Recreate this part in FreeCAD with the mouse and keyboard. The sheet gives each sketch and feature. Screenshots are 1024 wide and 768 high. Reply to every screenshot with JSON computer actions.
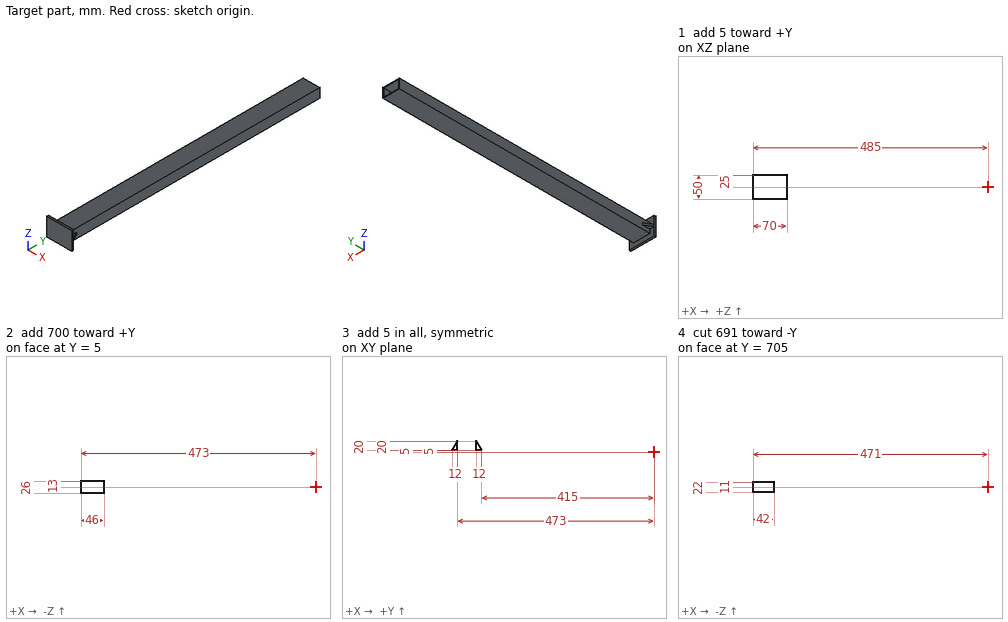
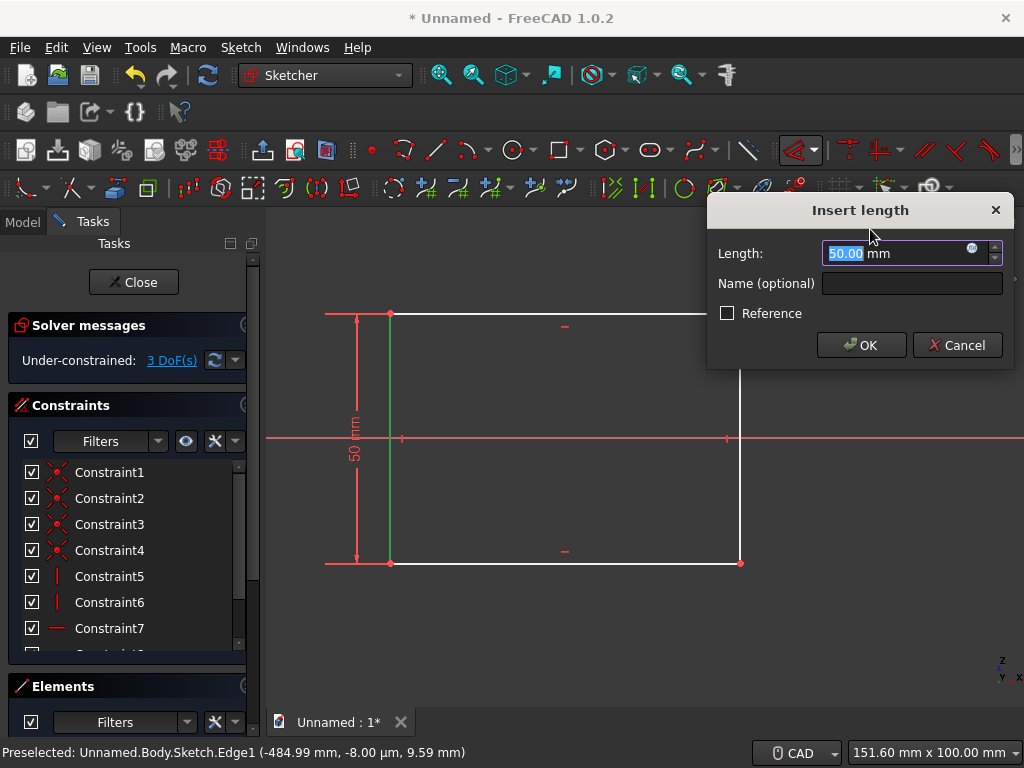
{"action": "type", "text": "50"}
{"action": "key", "text": "Return"}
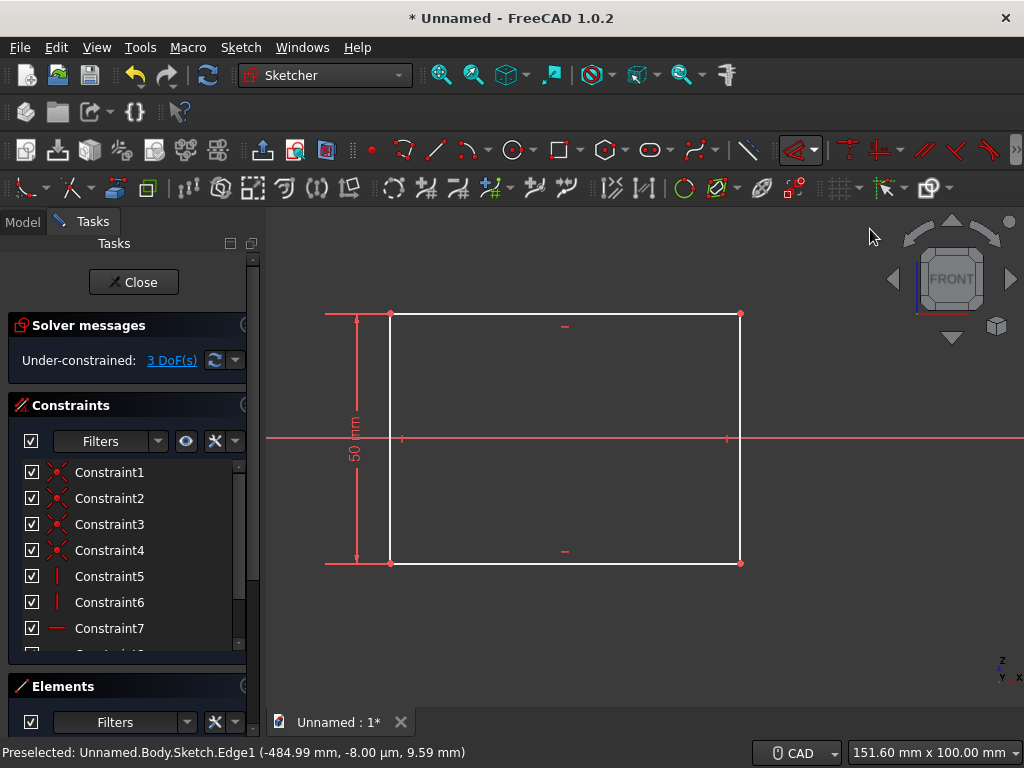
{"action": "left_click", "coordinate": [495, 564]}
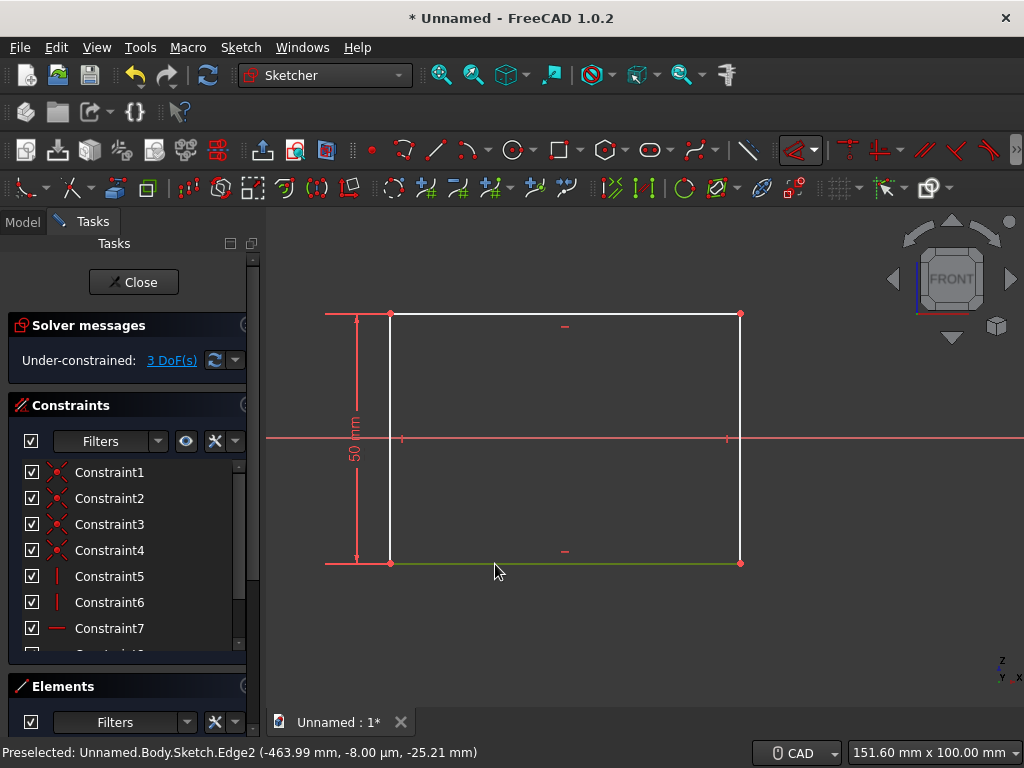
{"action": "key", "text": "l"}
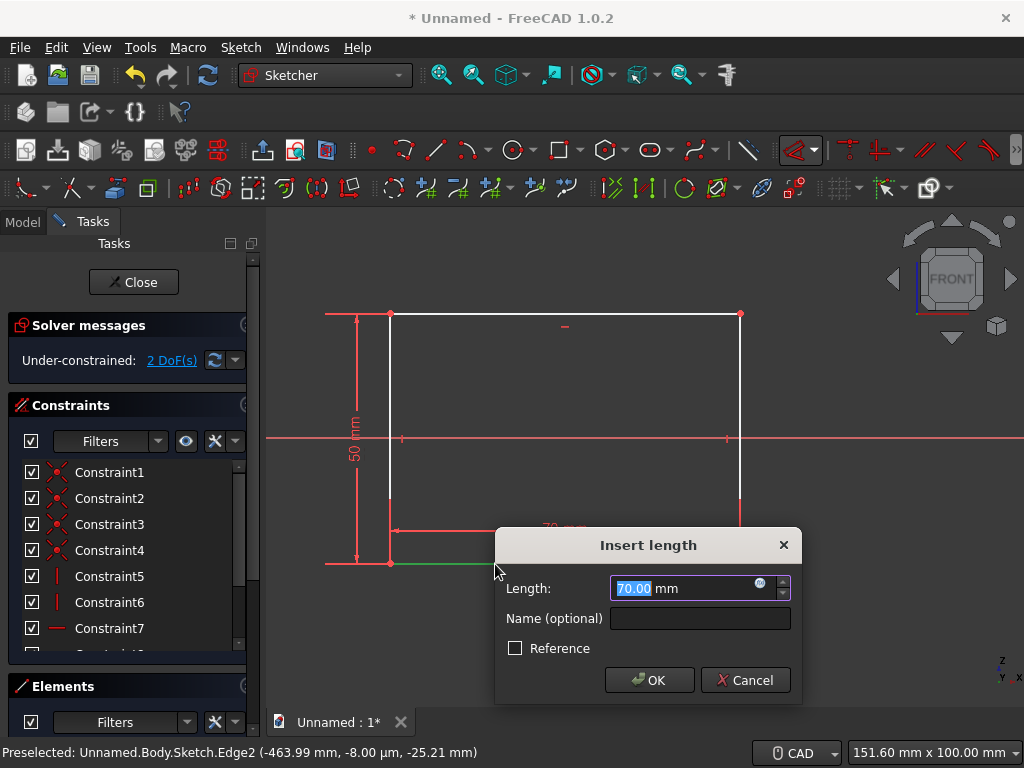
{"action": "type", "text": "70"}
{"action": "key", "text": "Return"}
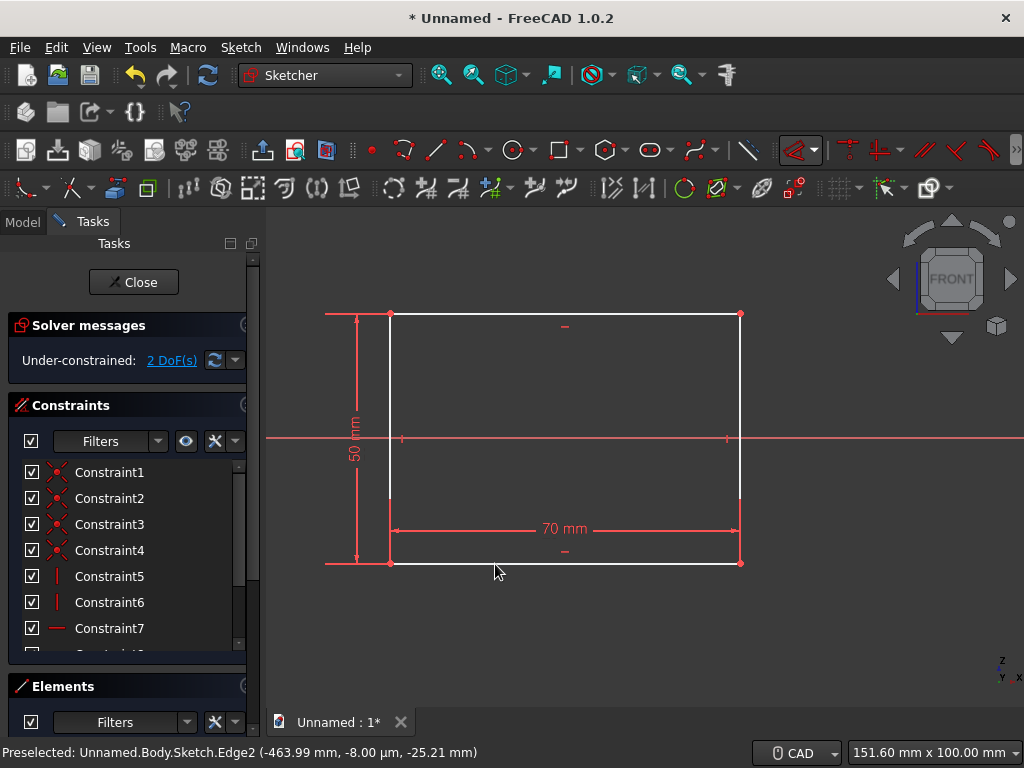
{"action": "left_click", "coordinate": [390, 314]}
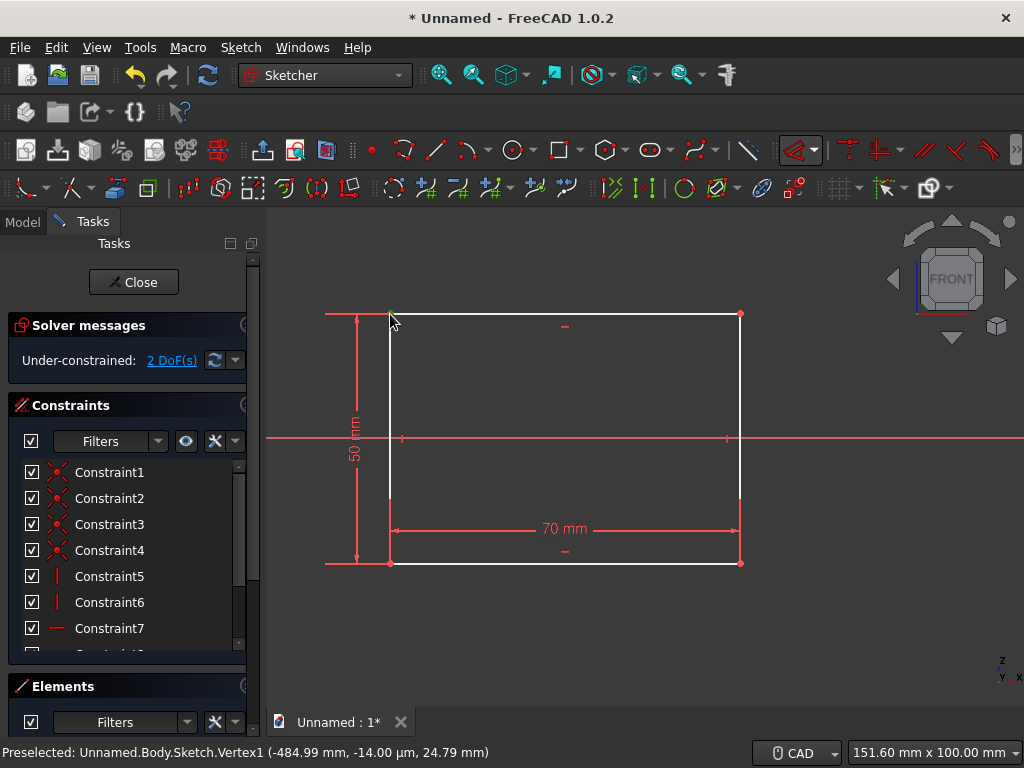
{"action": "left_click", "coordinate": [816, 150]}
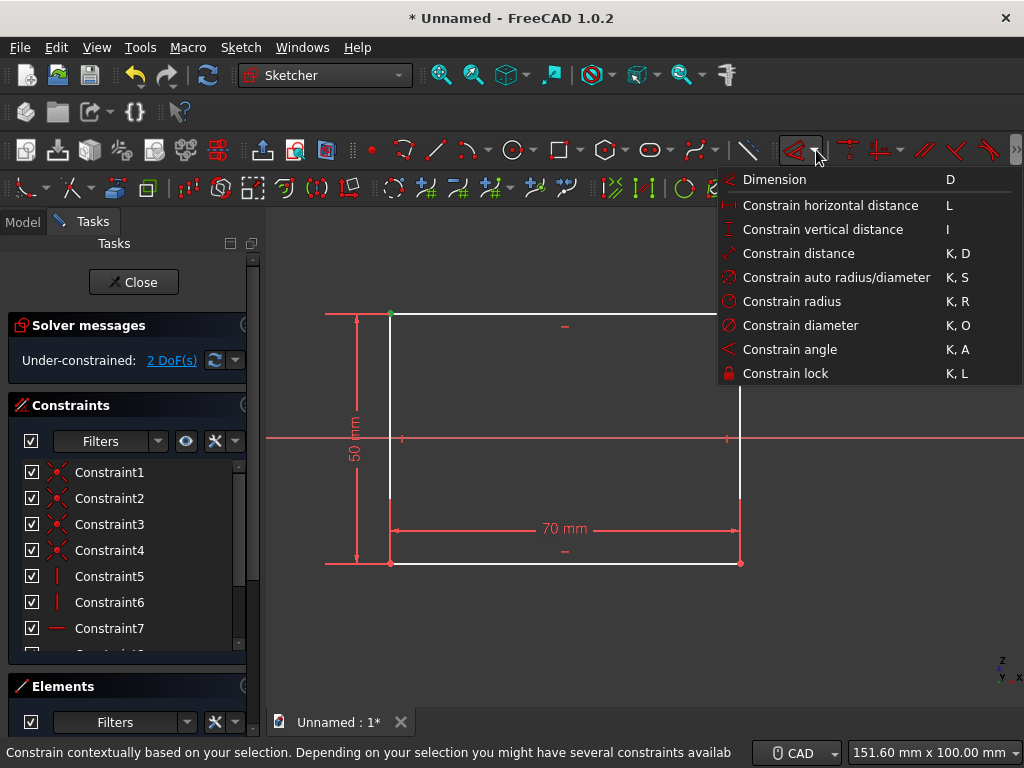
{"action": "left_click", "coordinate": [870, 229]}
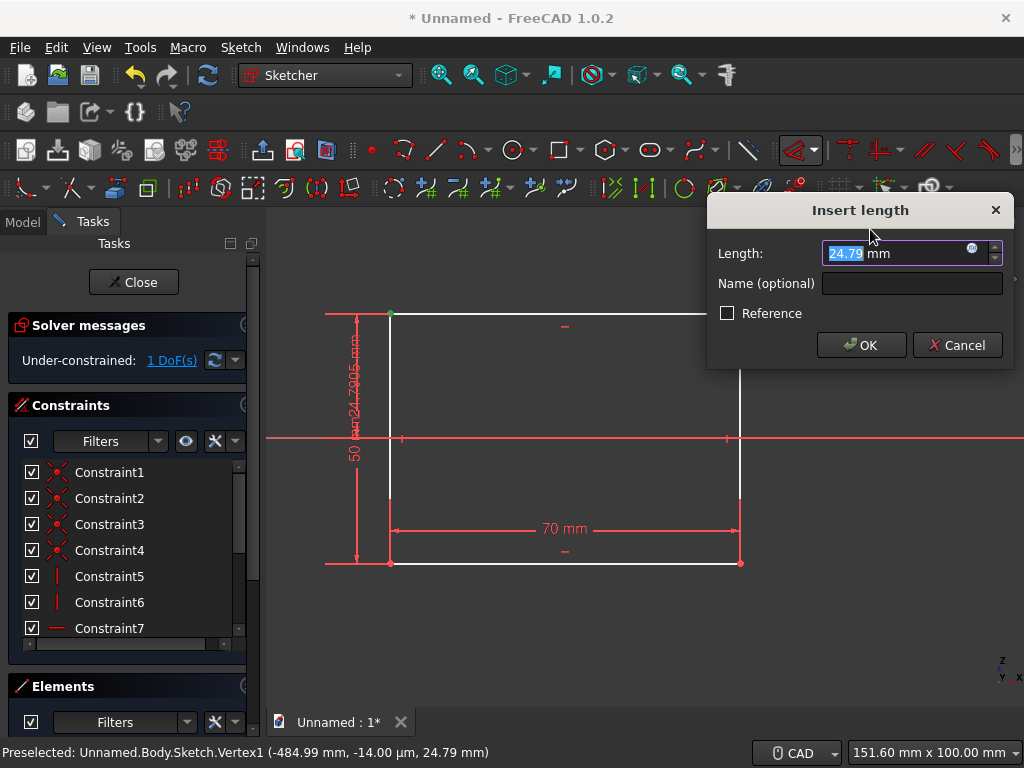
{"action": "type", "text": "25"}
{"action": "key", "text": "Return"}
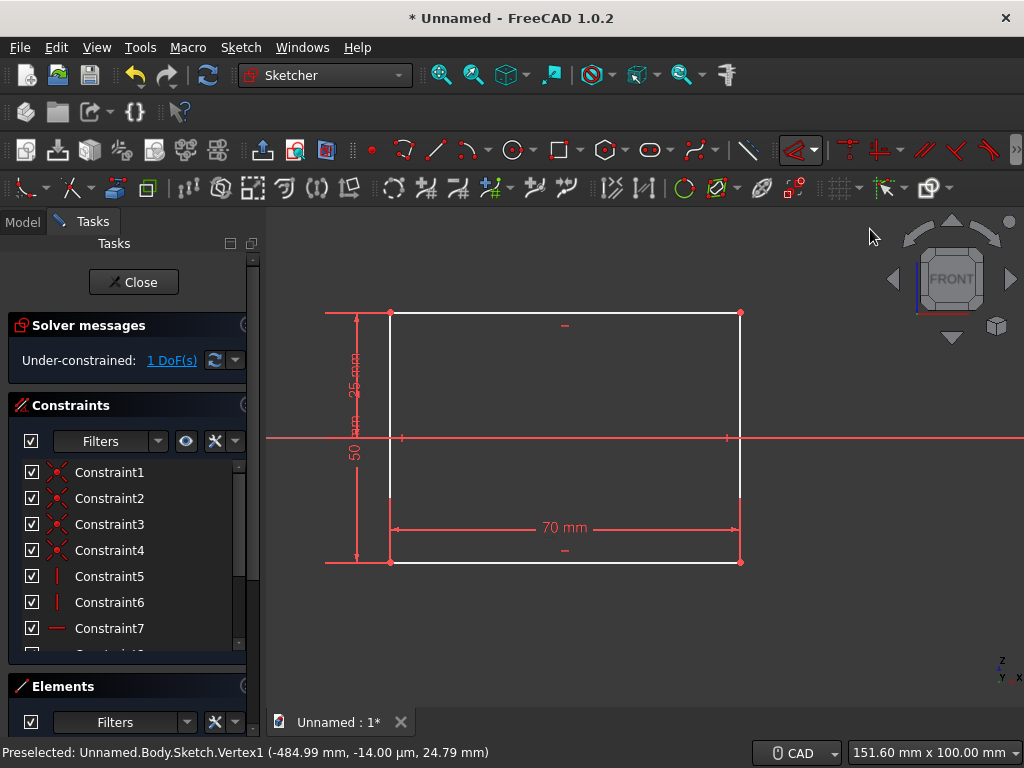
{"action": "left_click", "coordinate": [390, 313]}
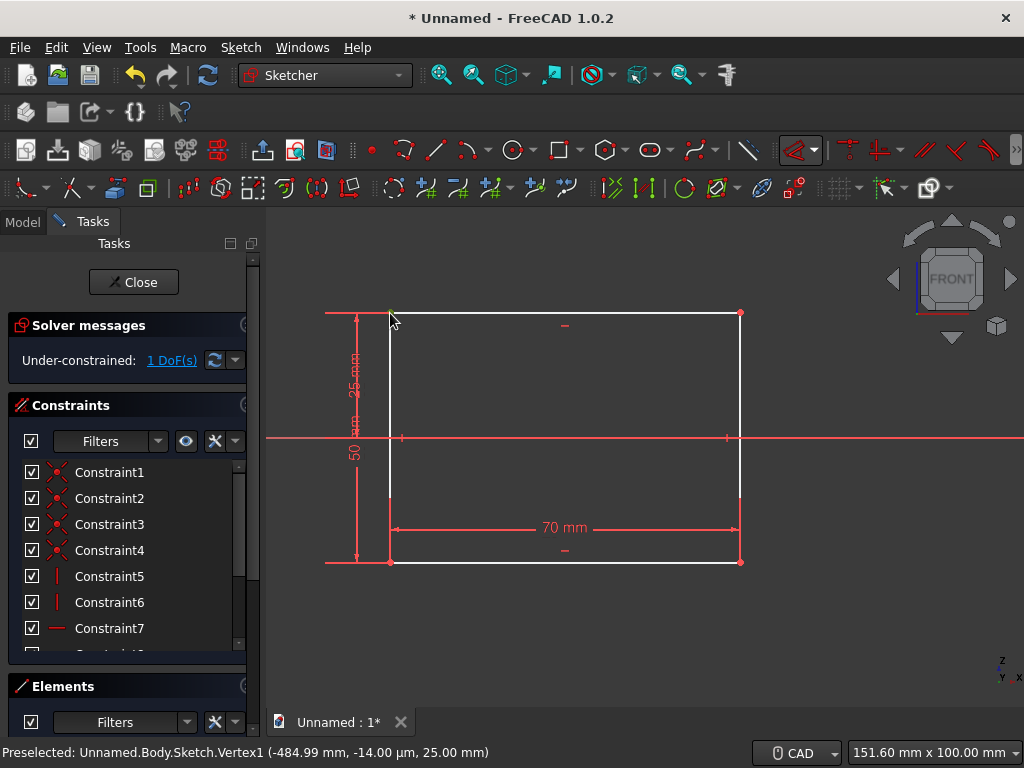
{"action": "key", "text": "l"}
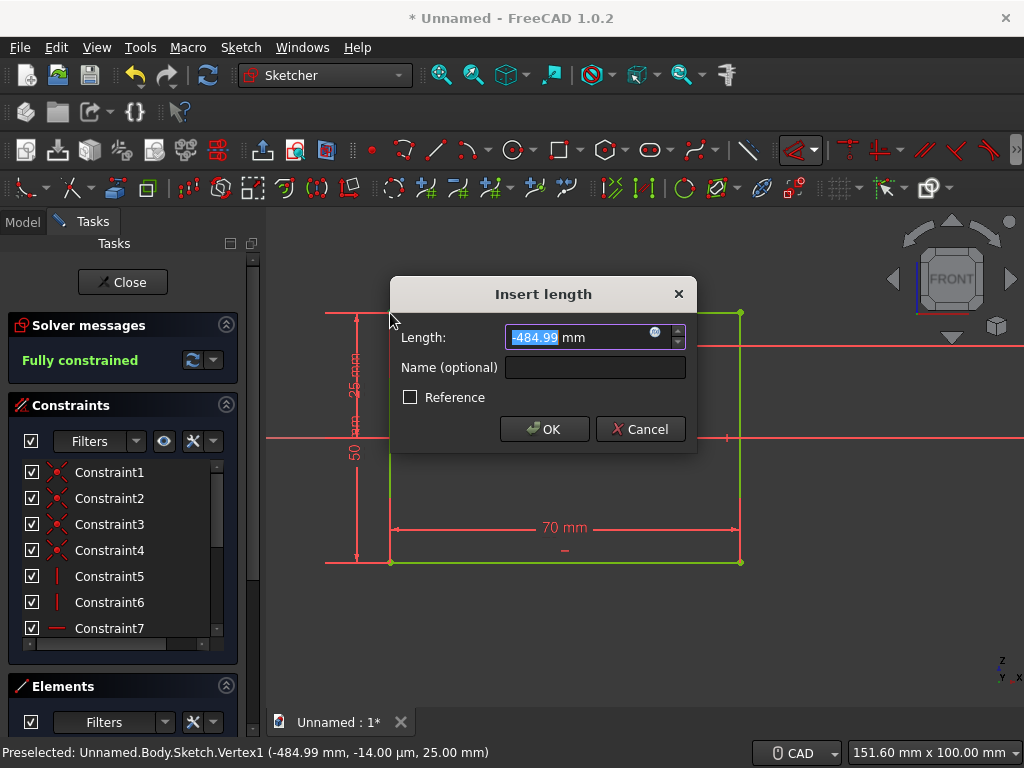
{"action": "type", "text": "-485"}
{"action": "key", "text": "Return"}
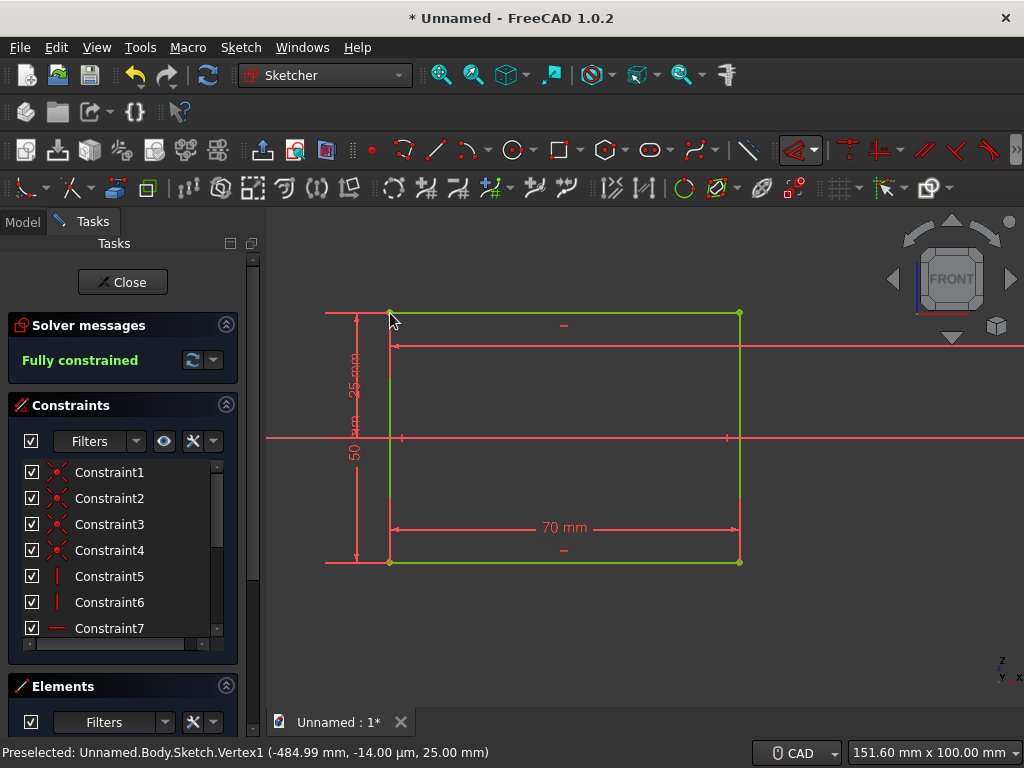
{"action": "left_click", "coordinate": [123, 282]}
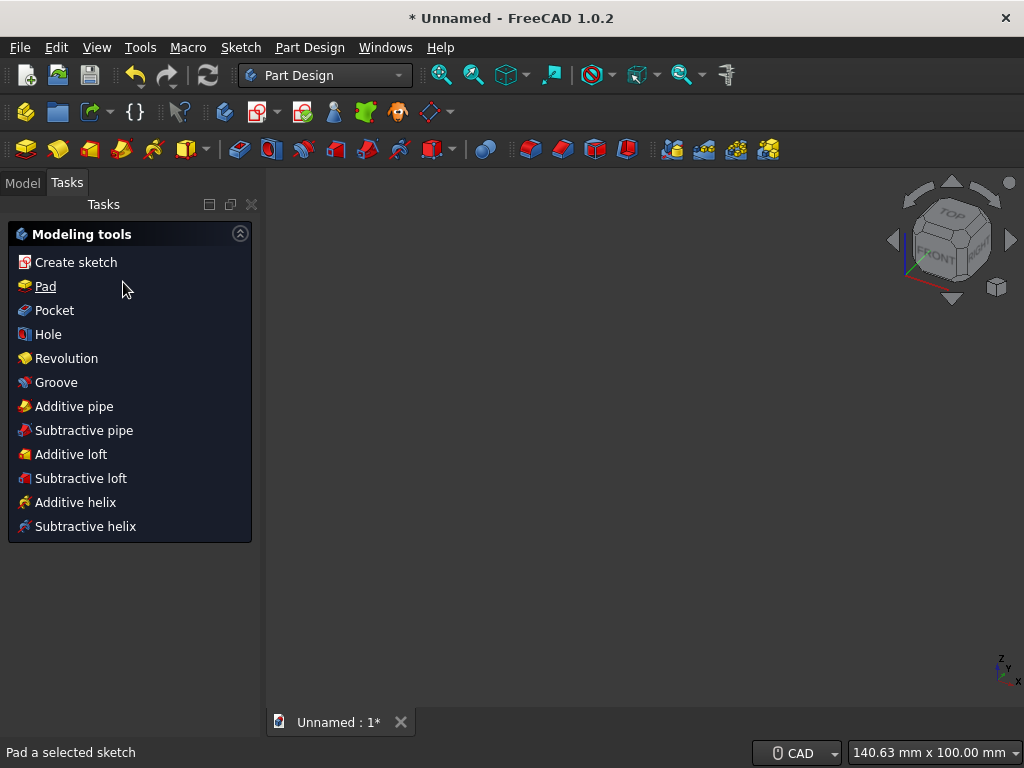
{"action": "left_click", "coordinate": [26, 150]}